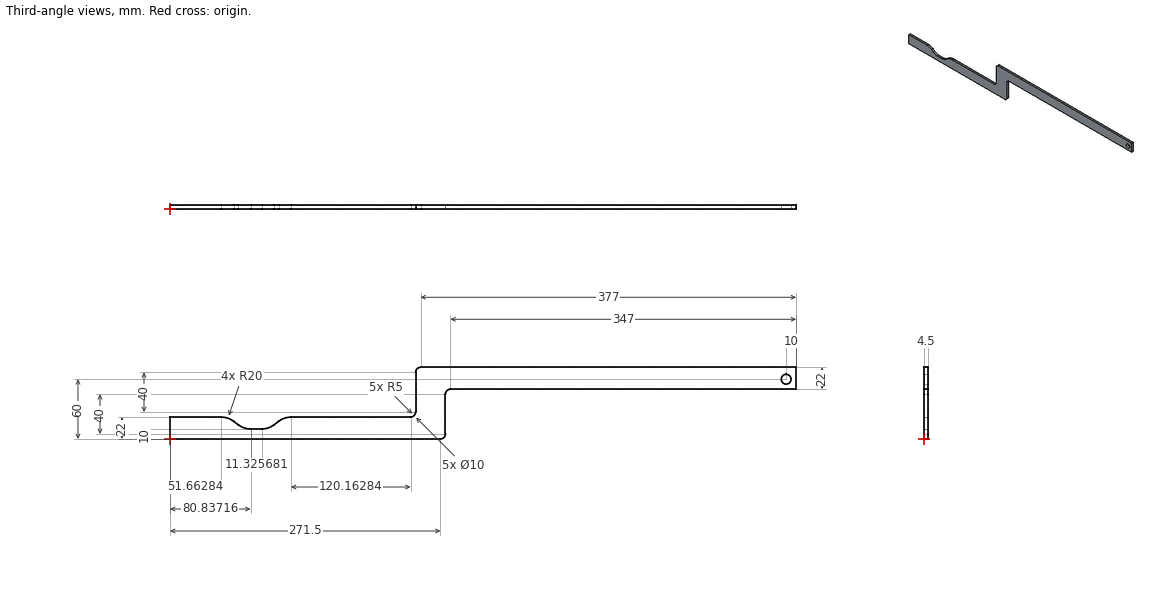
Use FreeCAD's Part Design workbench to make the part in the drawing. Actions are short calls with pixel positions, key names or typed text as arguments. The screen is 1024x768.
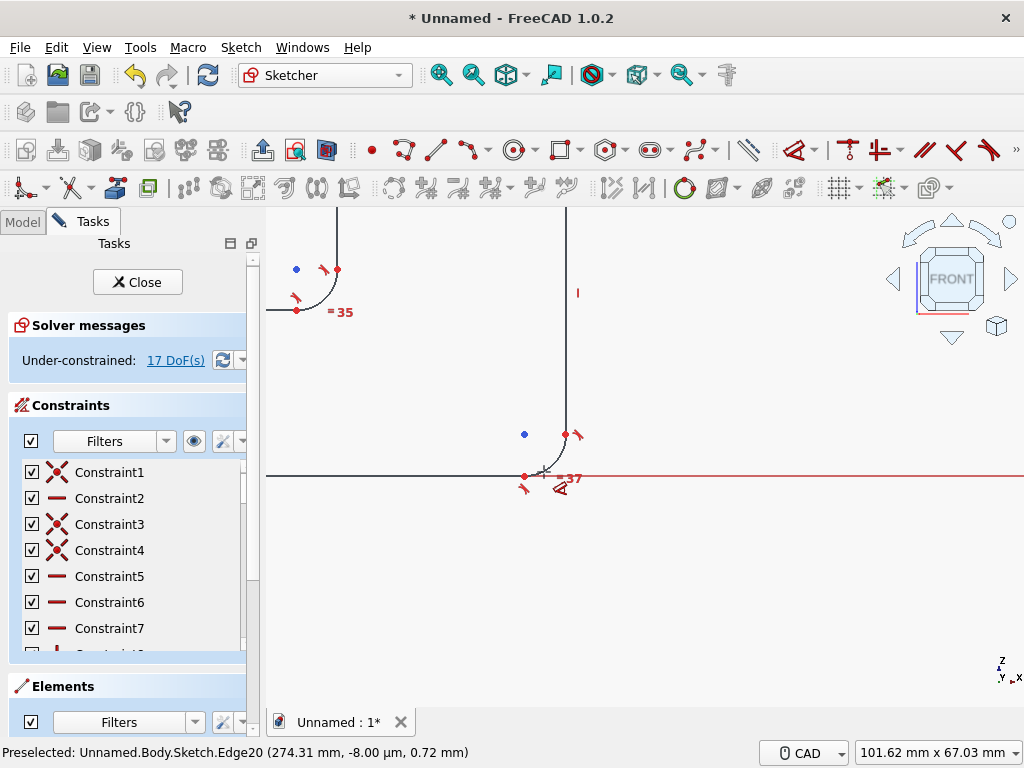
scroll(550, 482, down, 12)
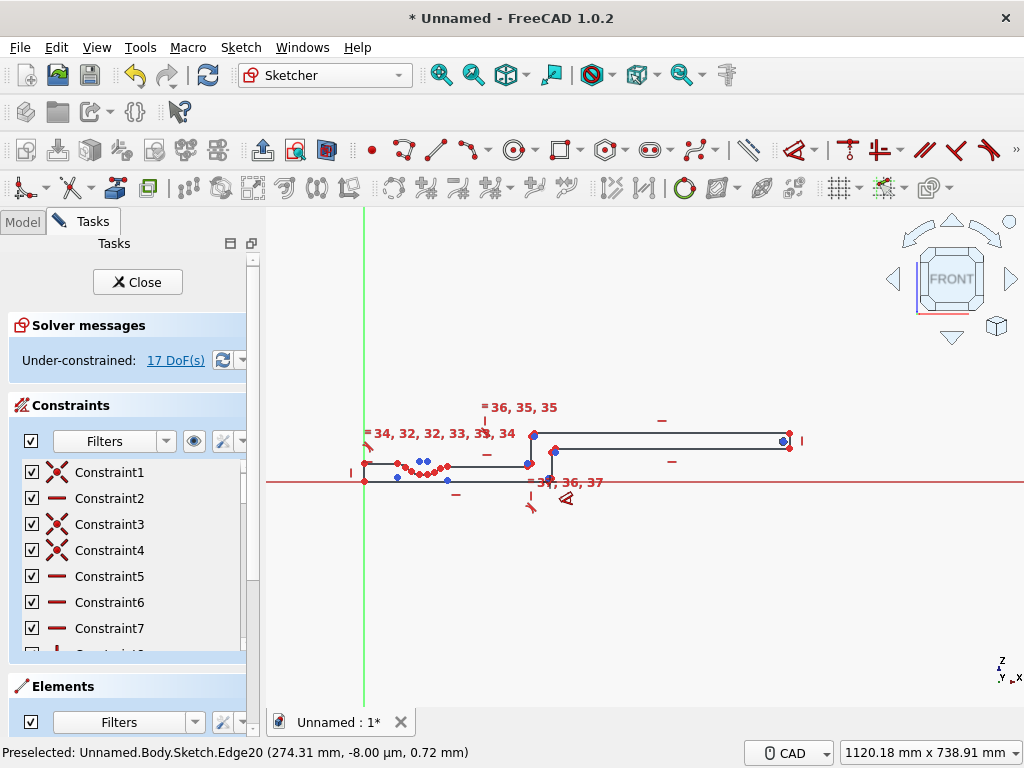
scroll(403, 465, up, 8)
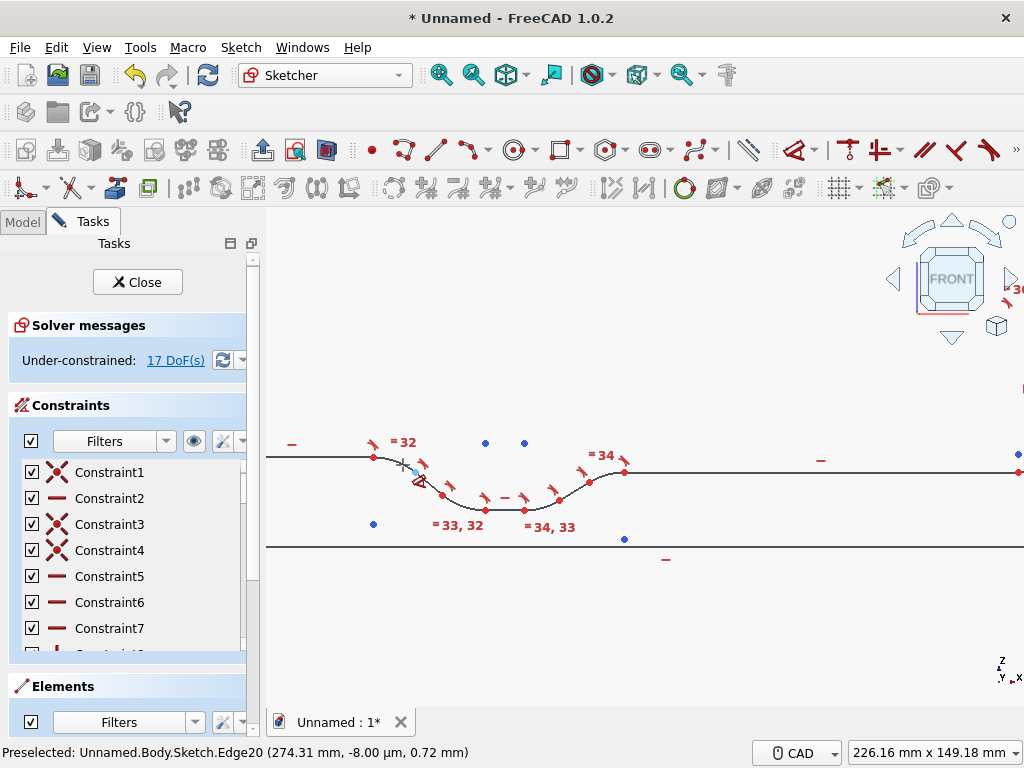
click(404, 465)
click(419, 437)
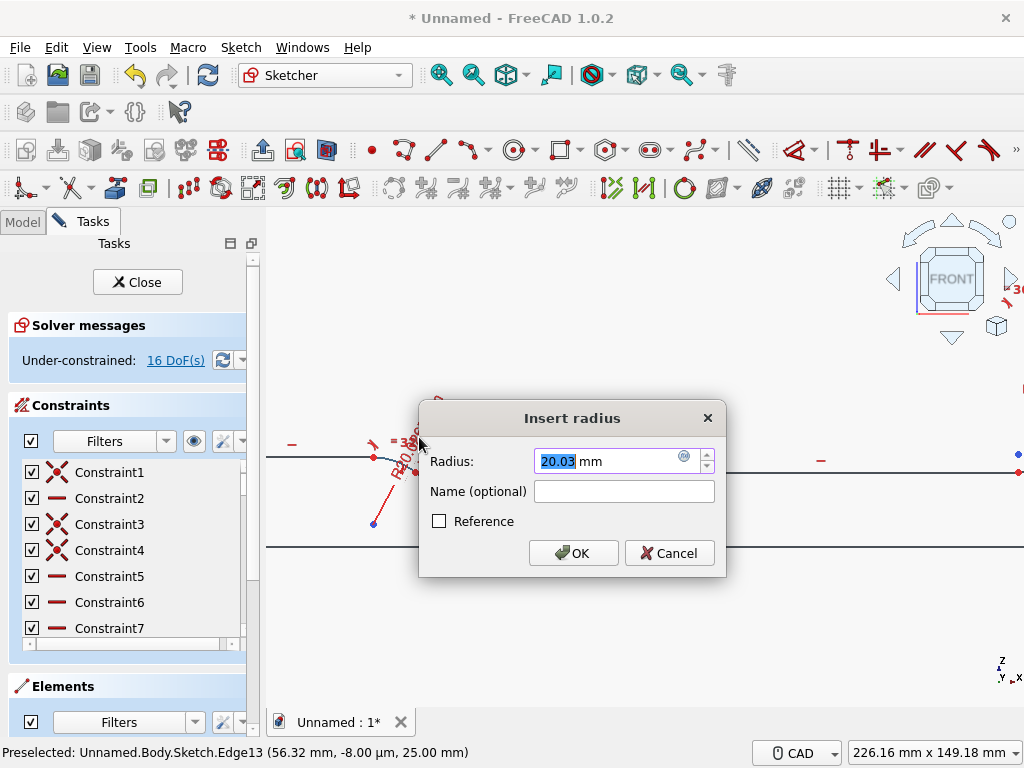
text(20)
key(Return)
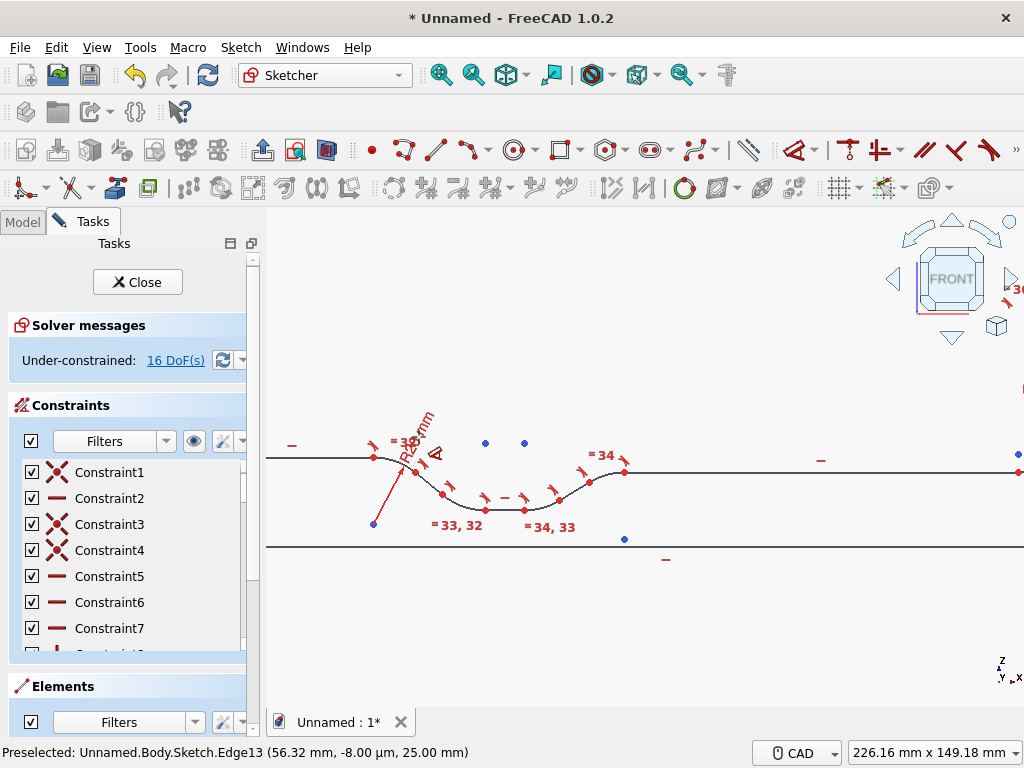
scroll(402, 465, down, 8)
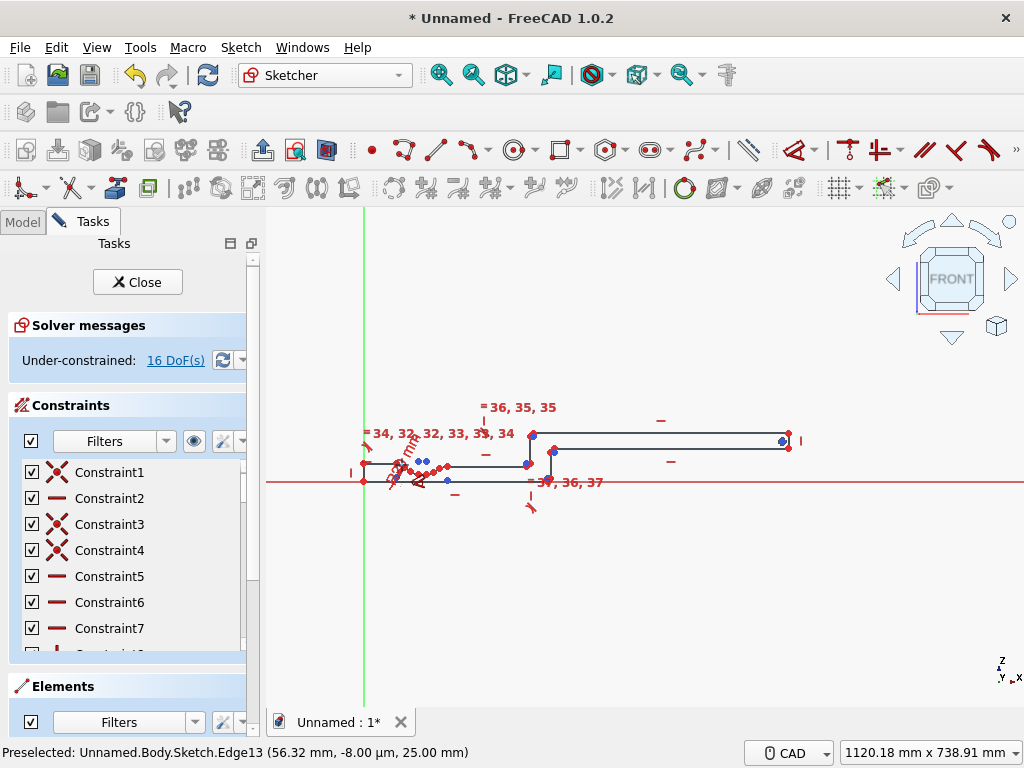
scroll(529, 466, up, 13)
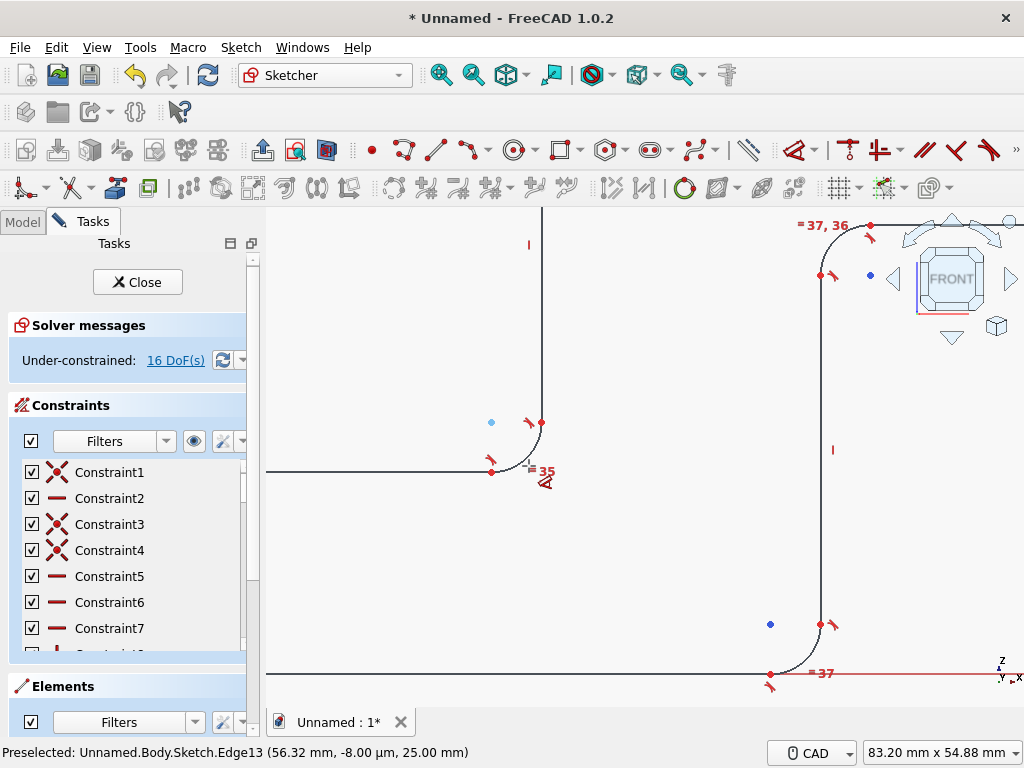
click(527, 458)
click(550, 481)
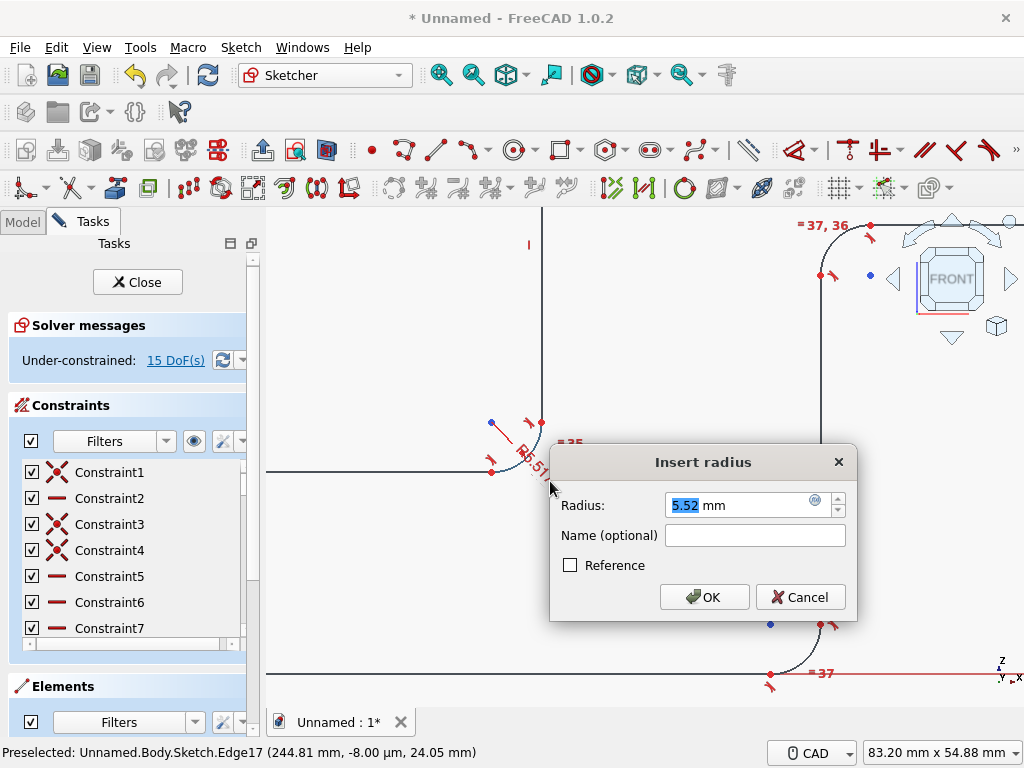
text(5)
key(Return)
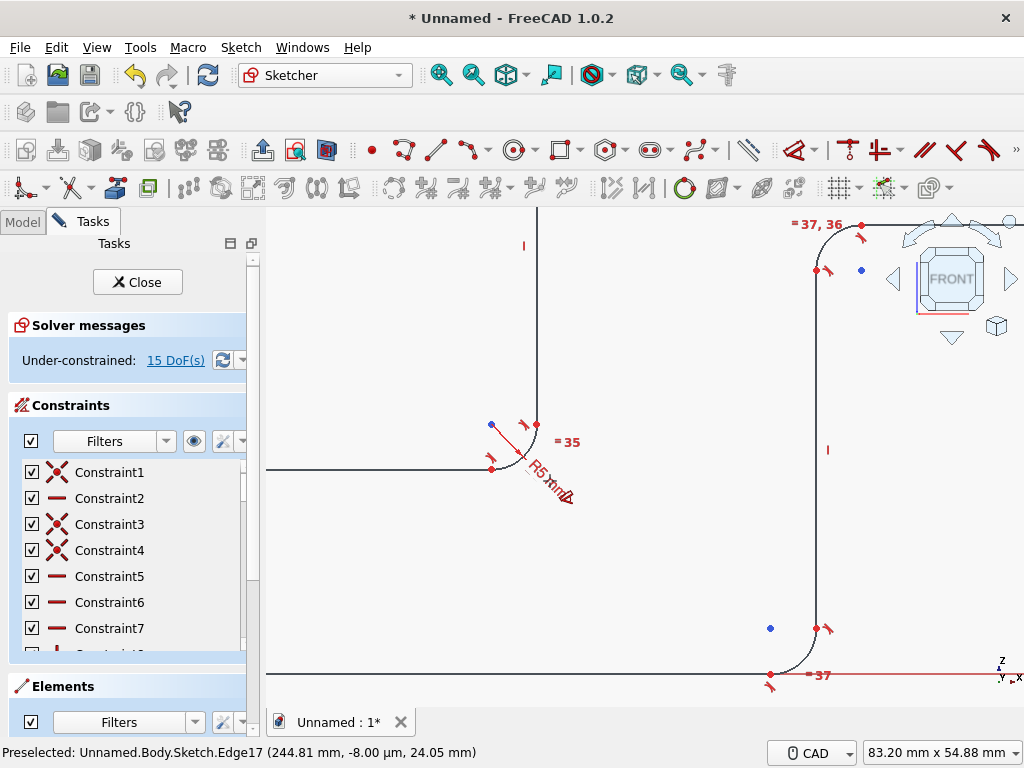
scroll(530, 466, down, 13)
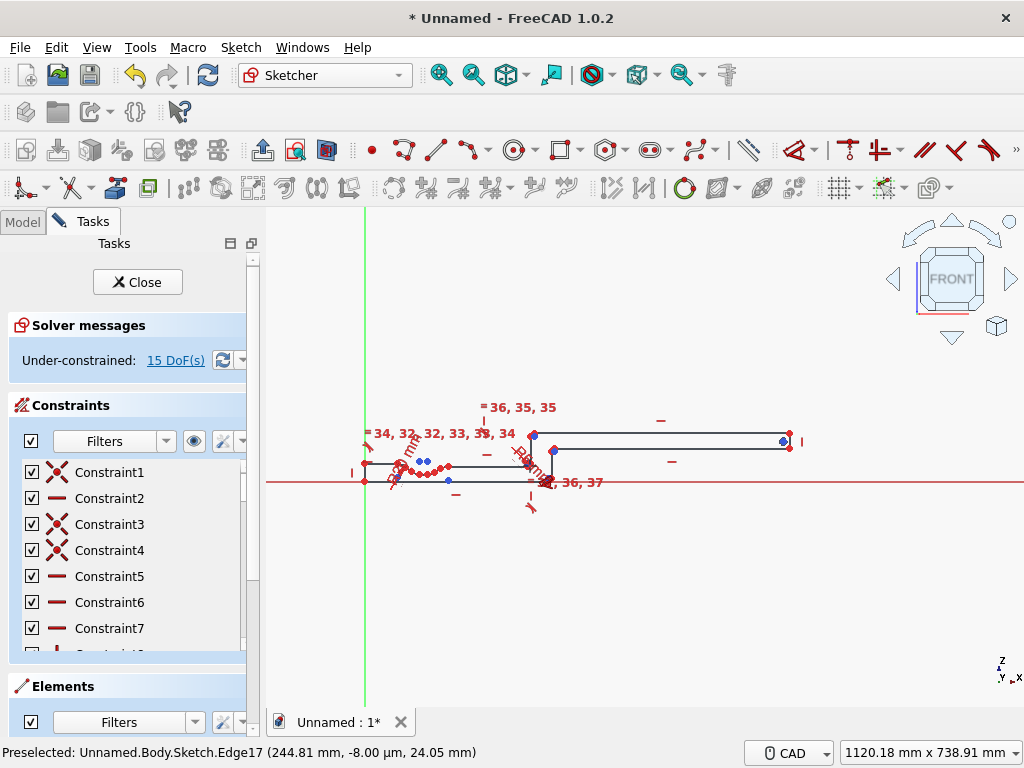
scroll(786, 439, up, 9)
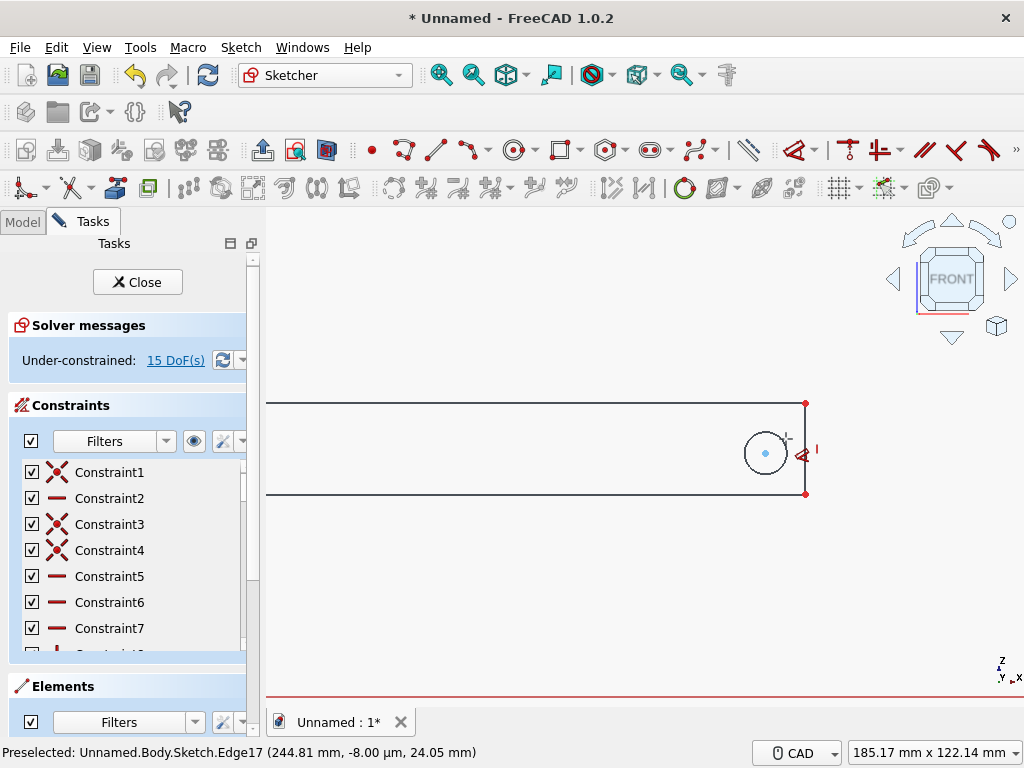
click(781, 438)
click(820, 399)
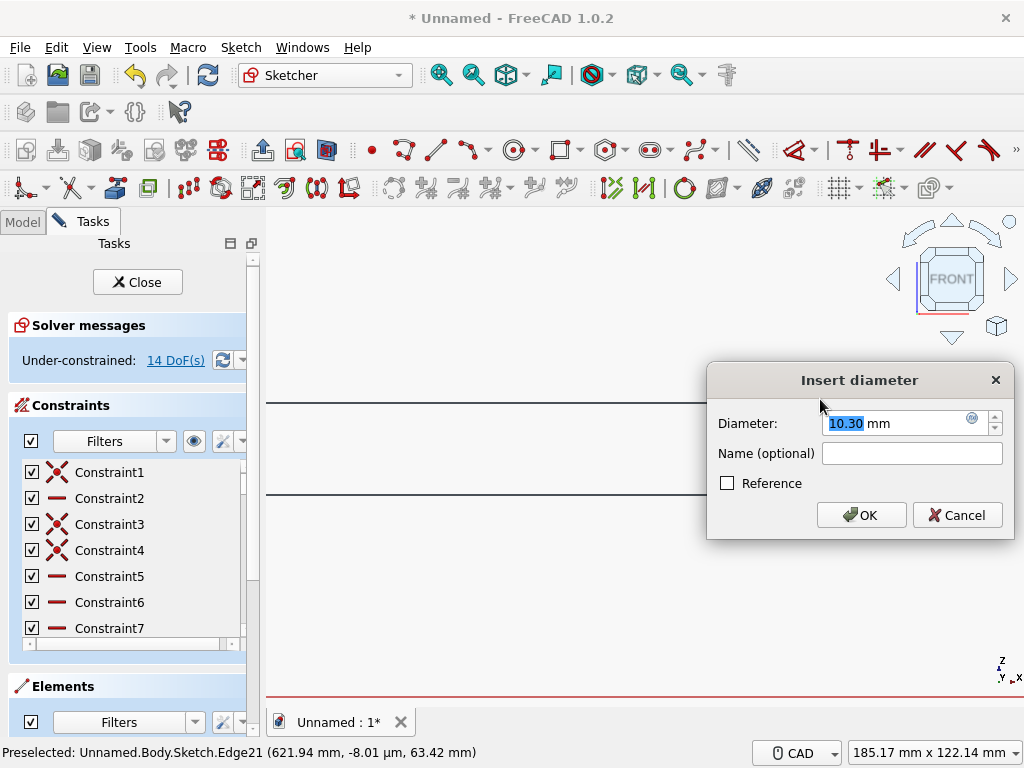
text(10)
key(Return)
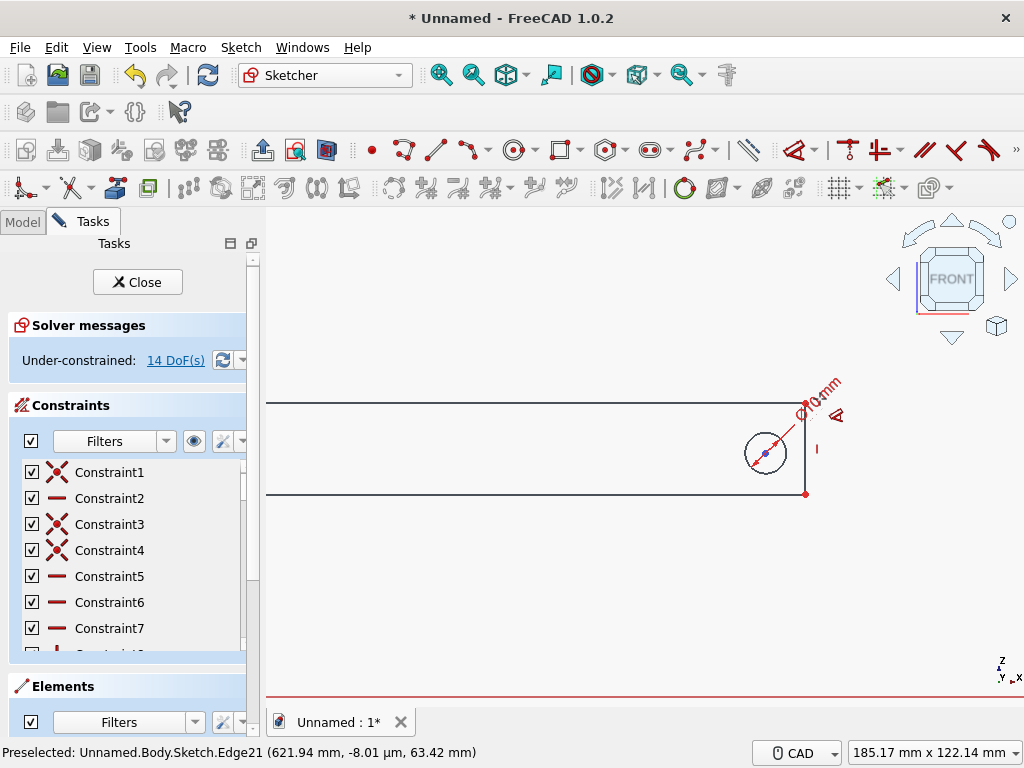
scroll(786, 439, down, 9)